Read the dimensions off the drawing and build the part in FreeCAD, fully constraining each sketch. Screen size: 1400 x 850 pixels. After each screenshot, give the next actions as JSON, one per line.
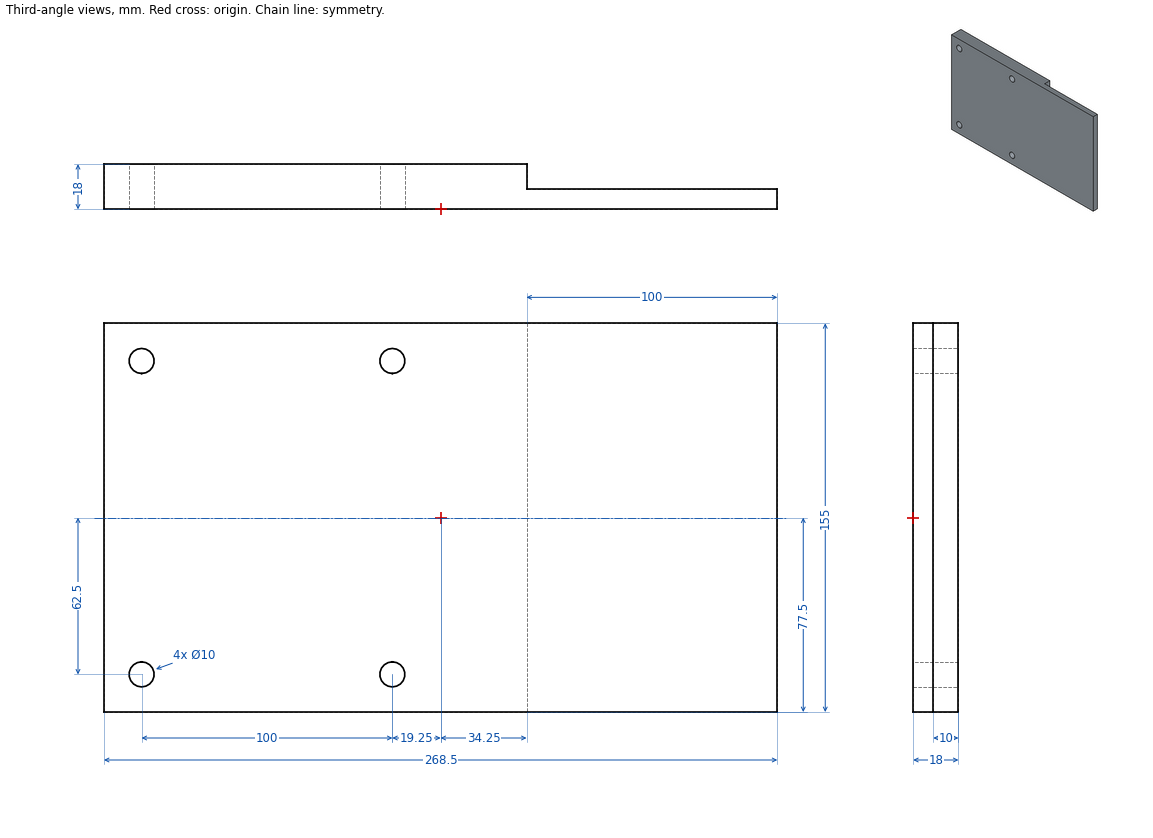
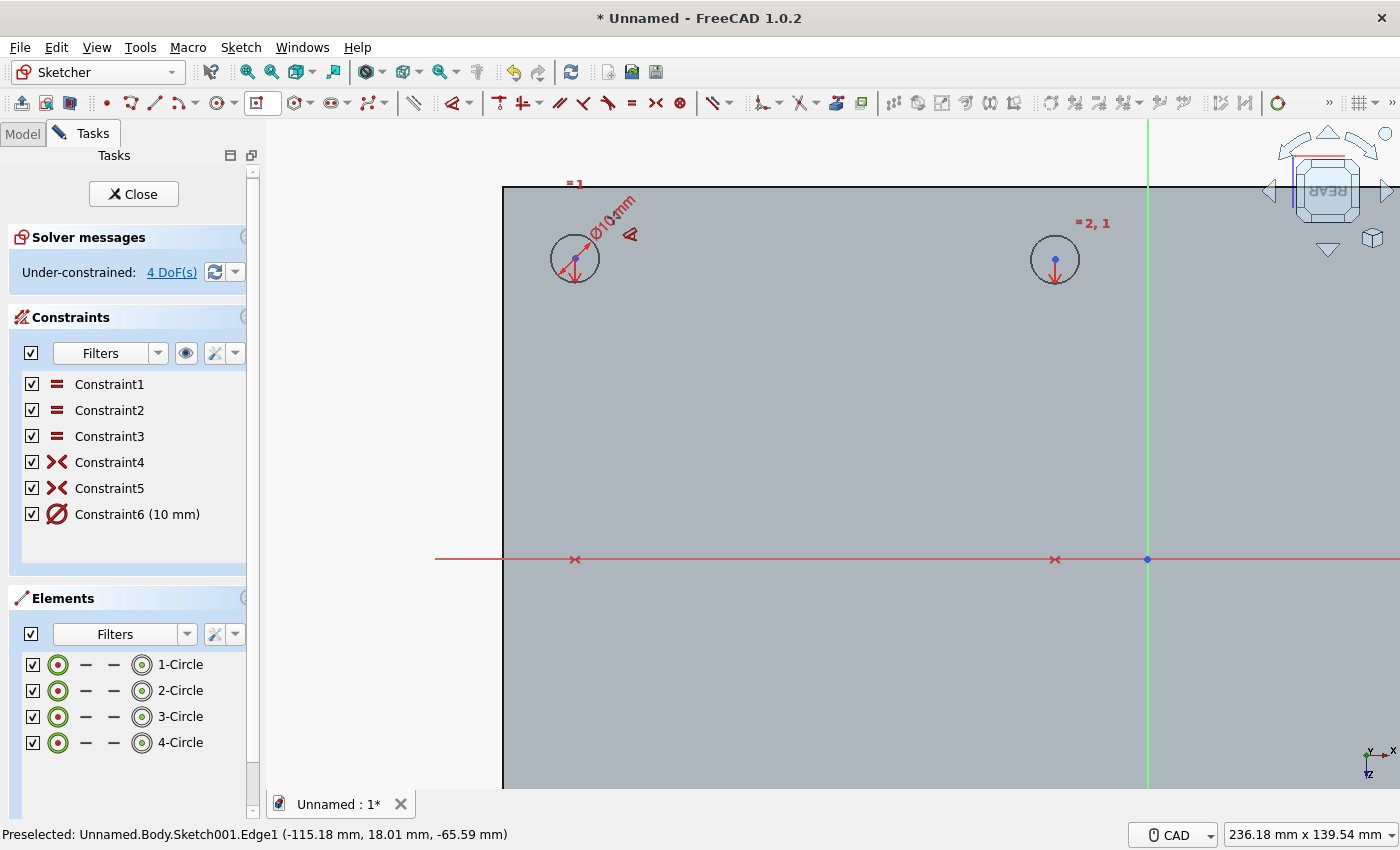
{"action": "left_click", "coordinate": [575, 259]}
{"action": "left_click", "coordinate": [1182, 409]}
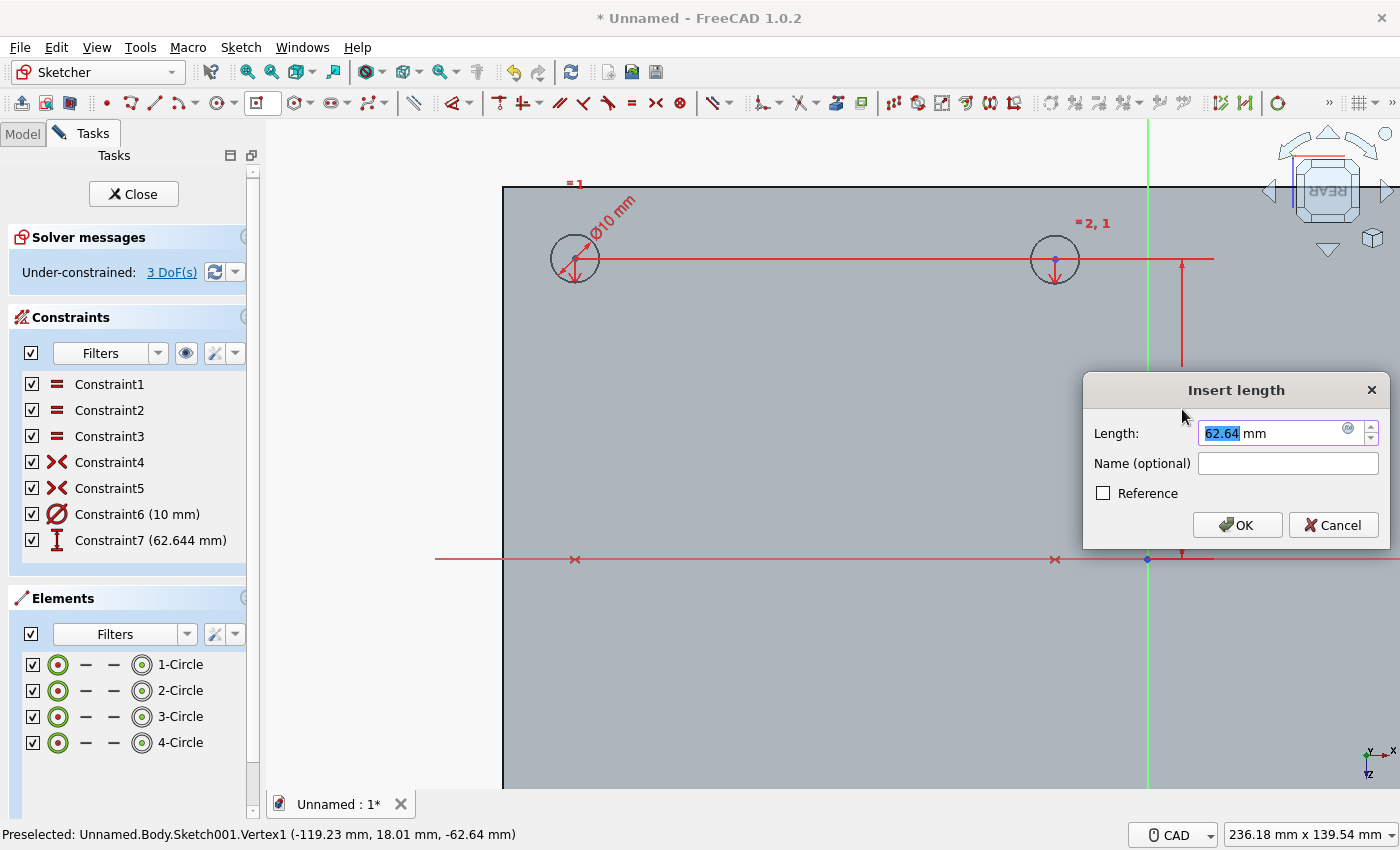
{"action": "type", "text": "62.5"}
{"action": "key", "text": "Return"}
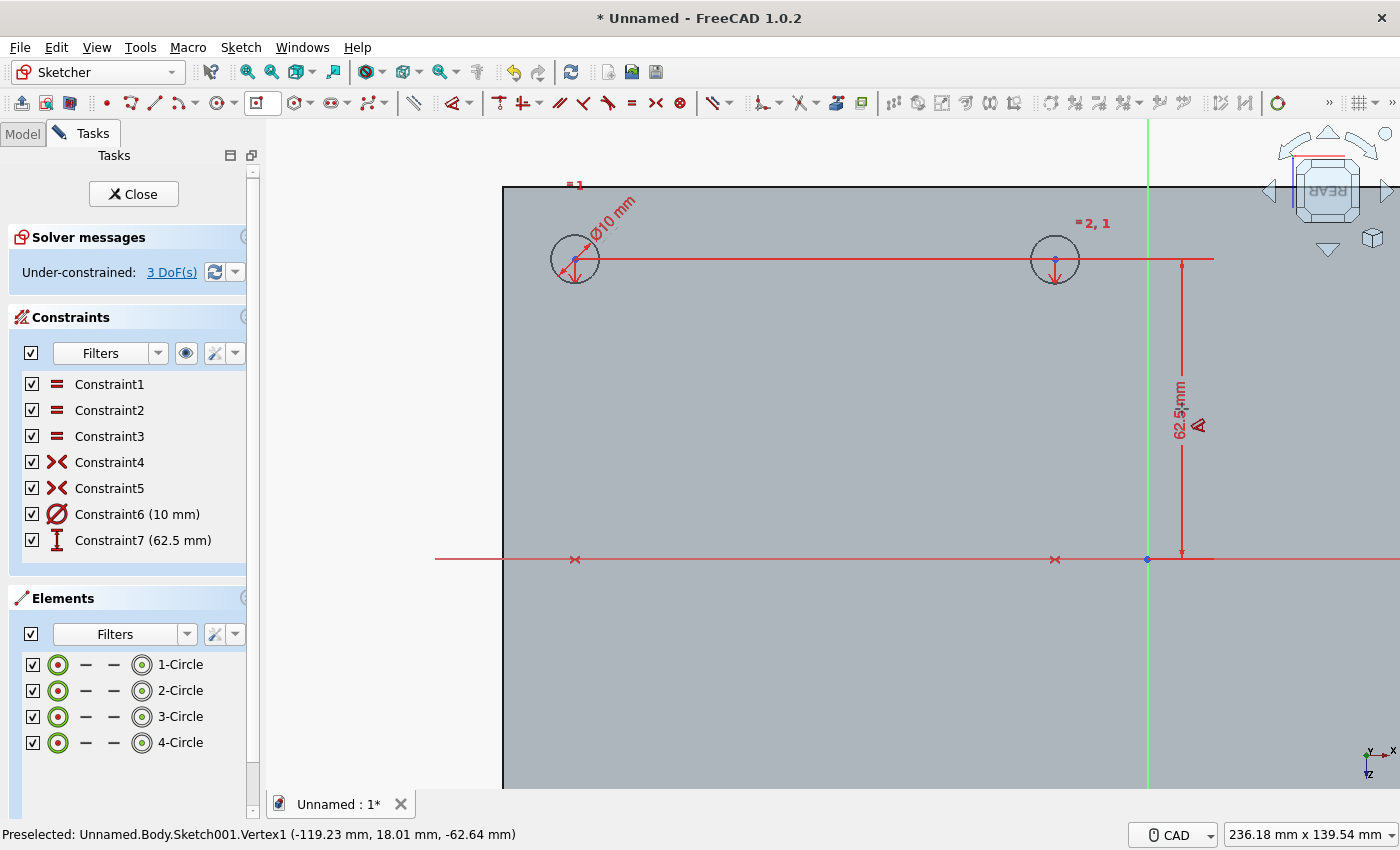
{"action": "left_click", "coordinate": [1055, 260]}
{"action": "left_click", "coordinate": [1182, 340]}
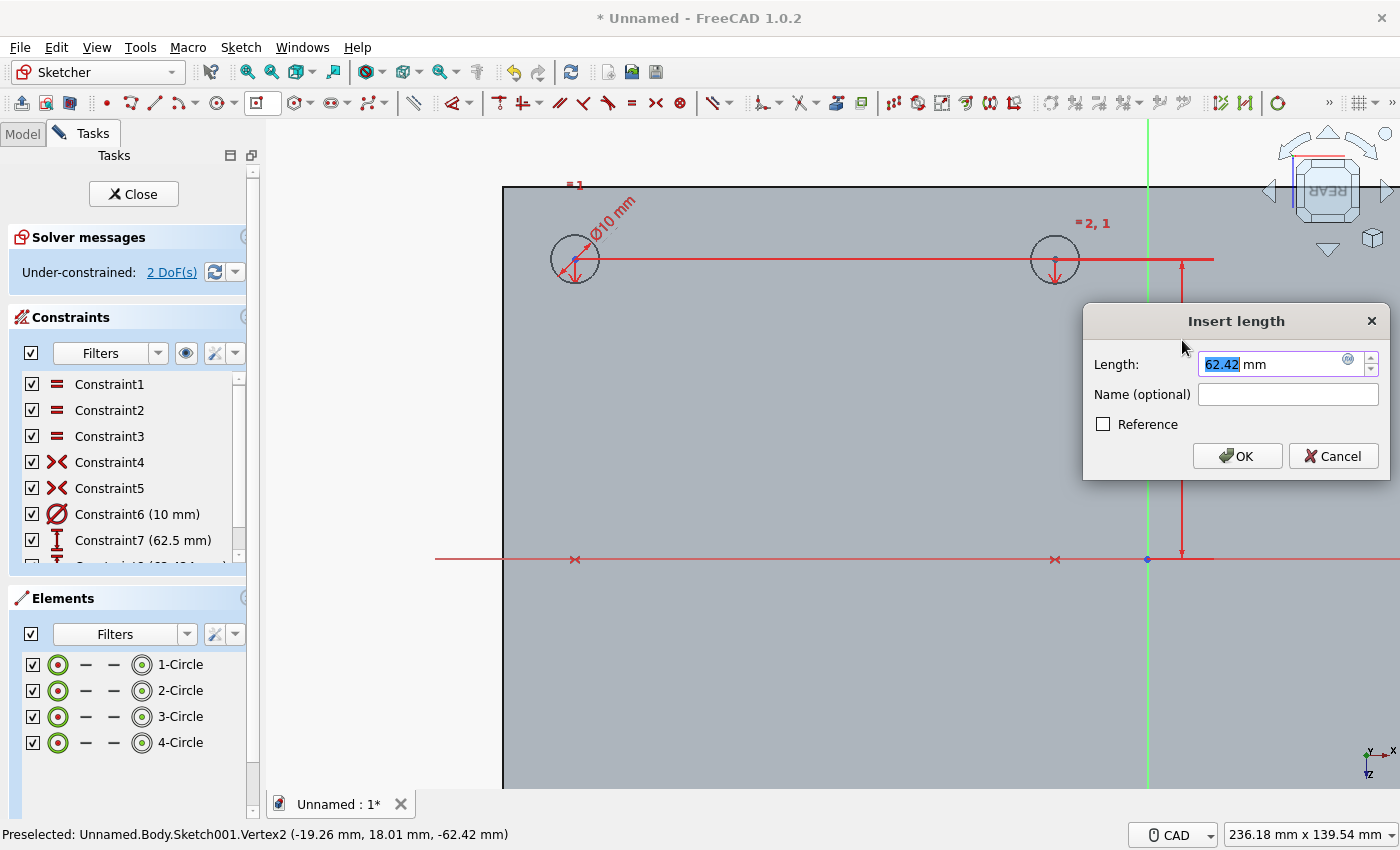
{"action": "type", "text": "62.5"}
{"action": "key", "text": "Return"}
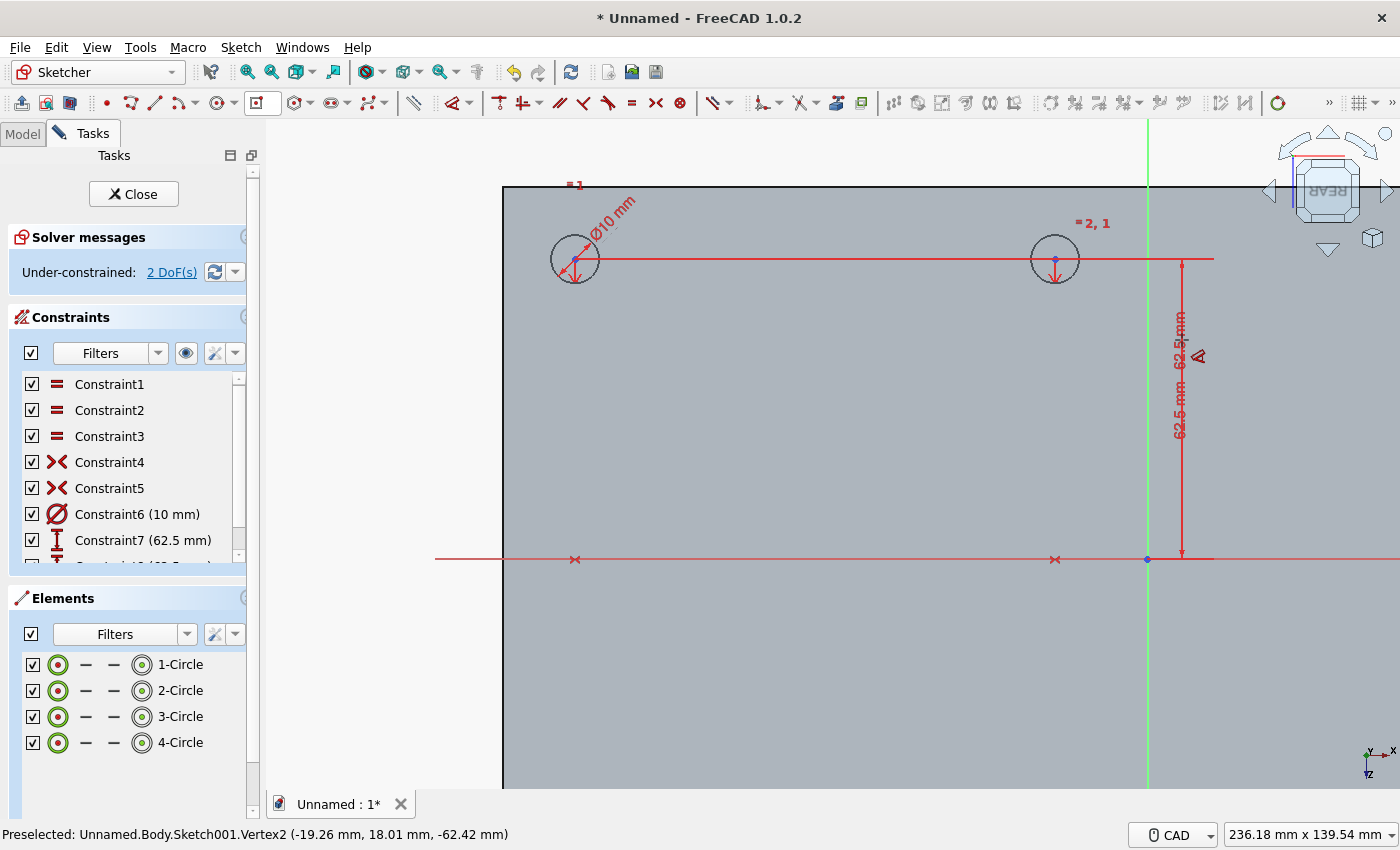
{"action": "left_click", "coordinate": [575, 259]}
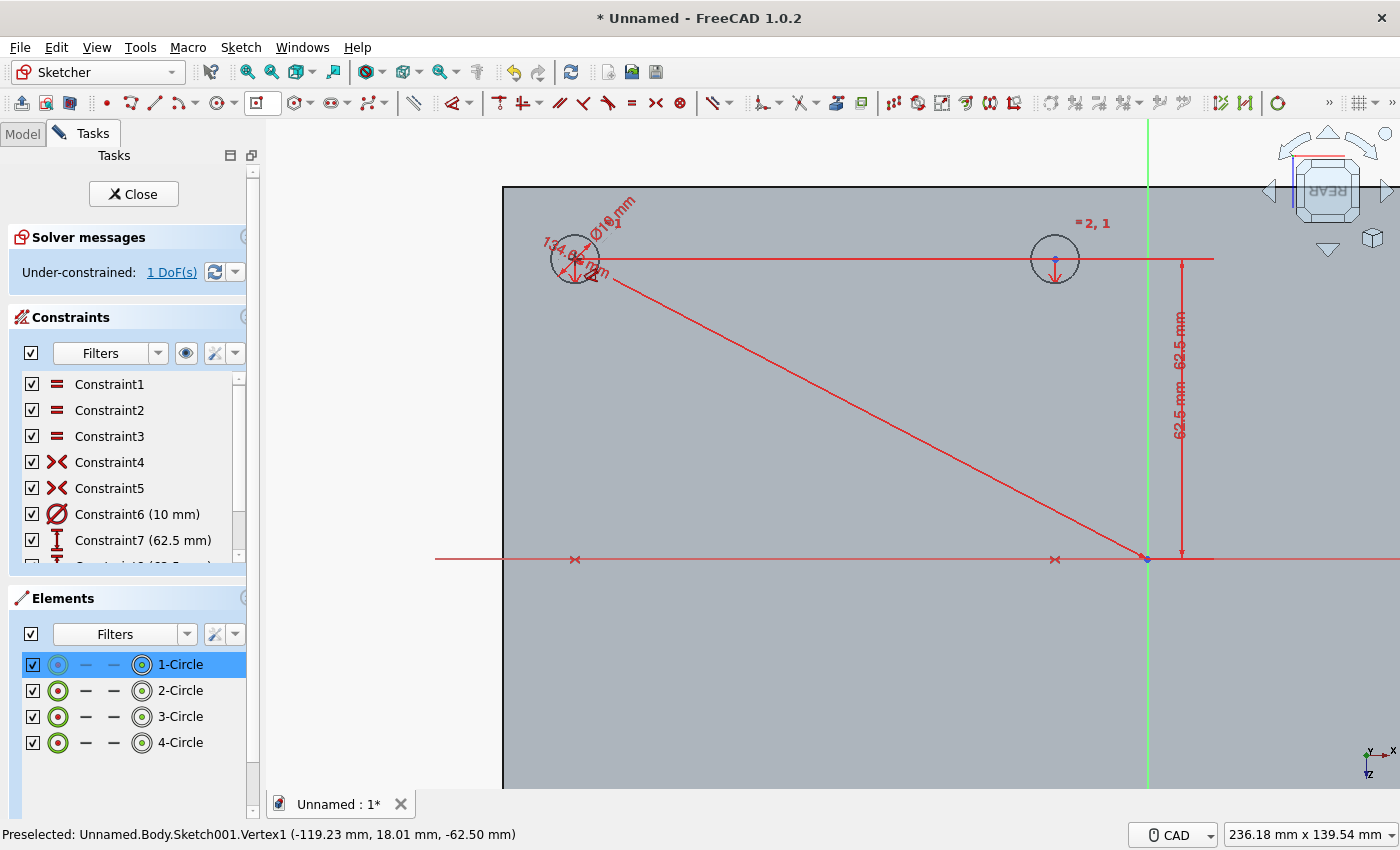
{"action": "left_click", "coordinate": [1055, 259]}
{"action": "left_click", "coordinate": [815, 225]}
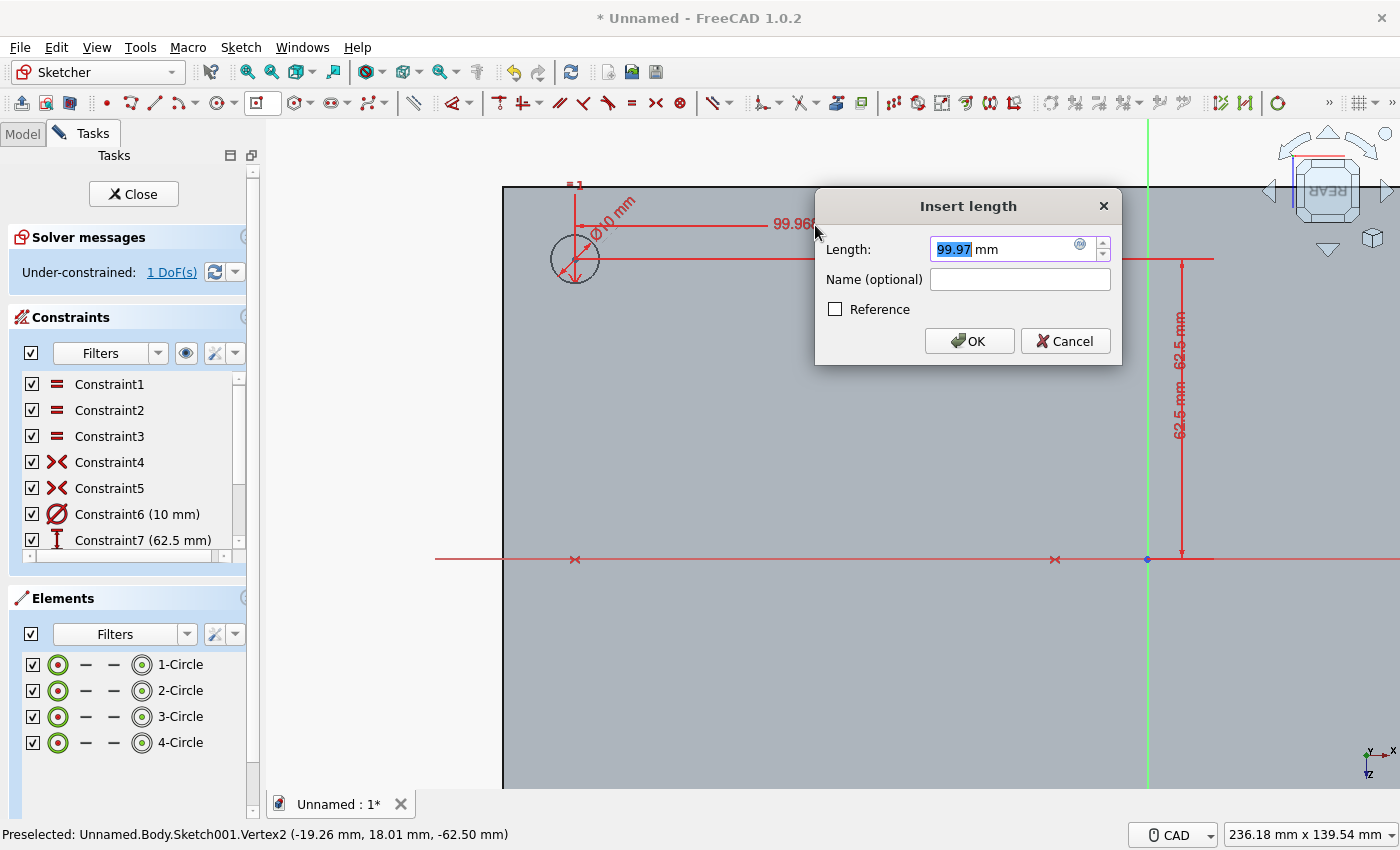
{"action": "type", "text": "100"}
{"action": "key", "text": "Return"}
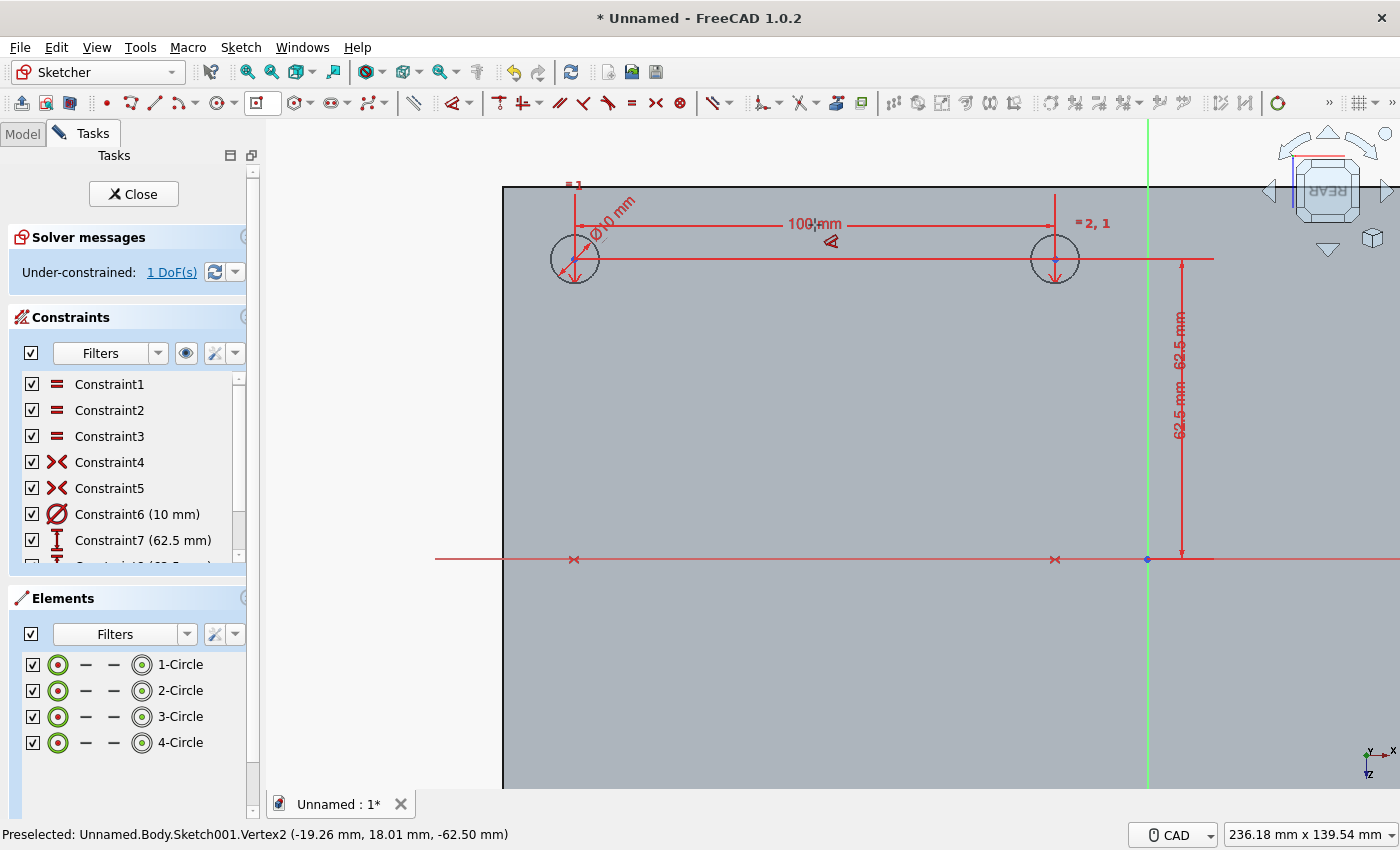
{"action": "left_click", "coordinate": [1055, 259]}
{"action": "left_click", "coordinate": [1101, 225]}